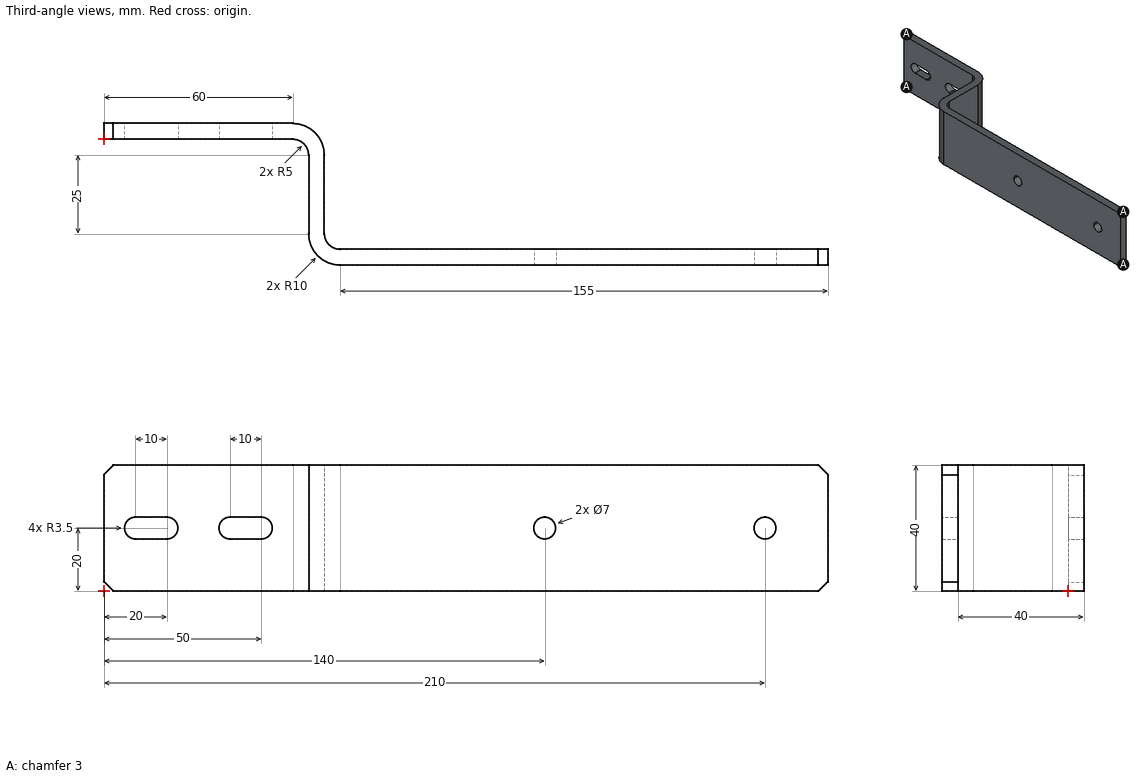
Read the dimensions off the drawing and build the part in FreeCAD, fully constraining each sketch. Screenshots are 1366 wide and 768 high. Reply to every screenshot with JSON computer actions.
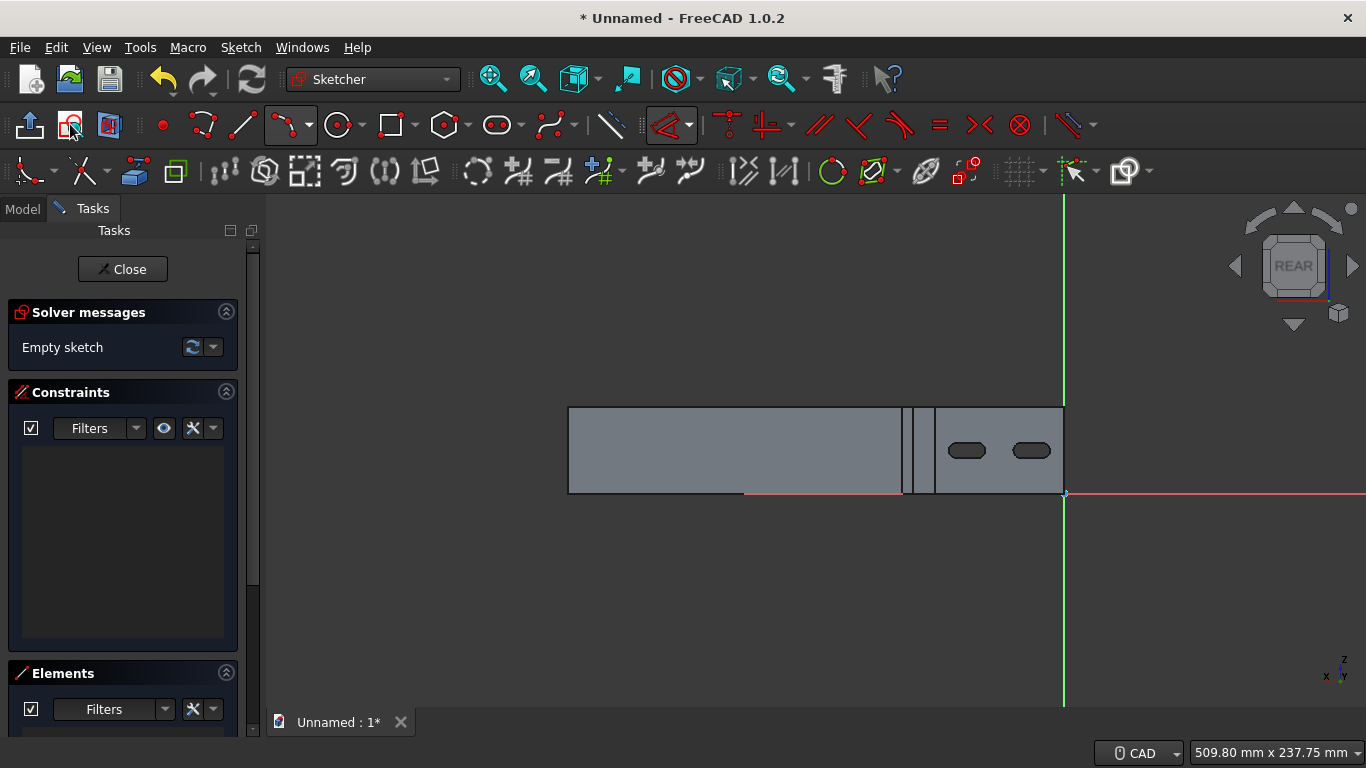
{"action": "left_click", "coordinate": [110, 126]}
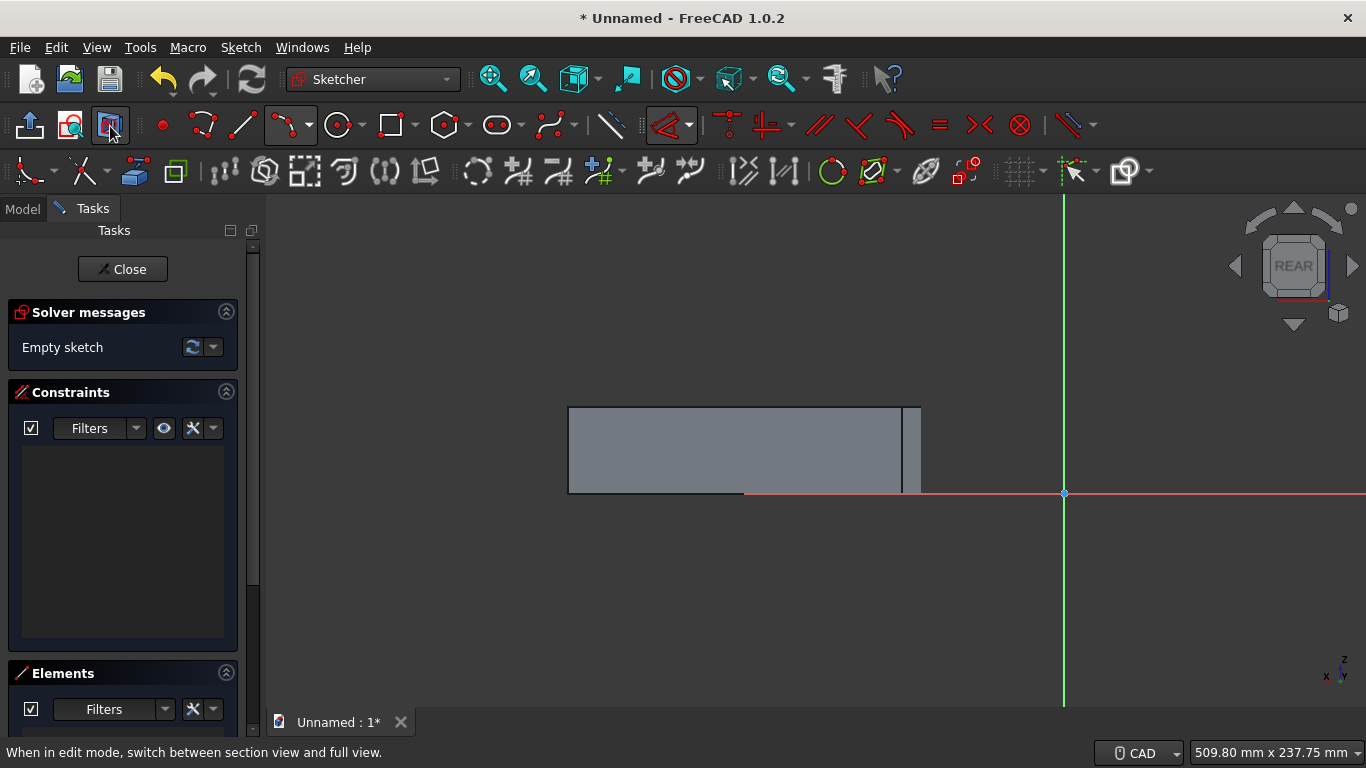
{"action": "scroll", "coordinate": [667, 451], "scroll_direction": "up", "scroll_amount": 7}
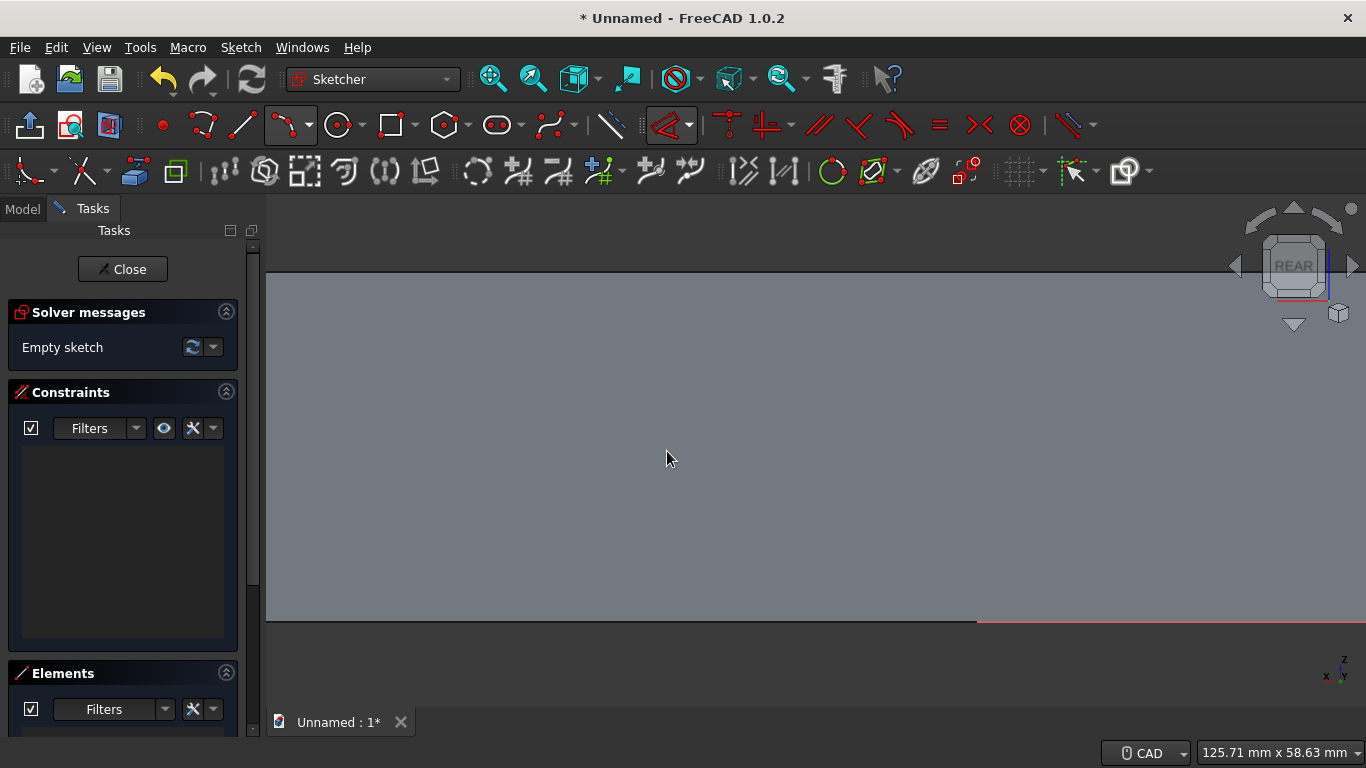
{"action": "left_click", "coordinate": [338, 126]}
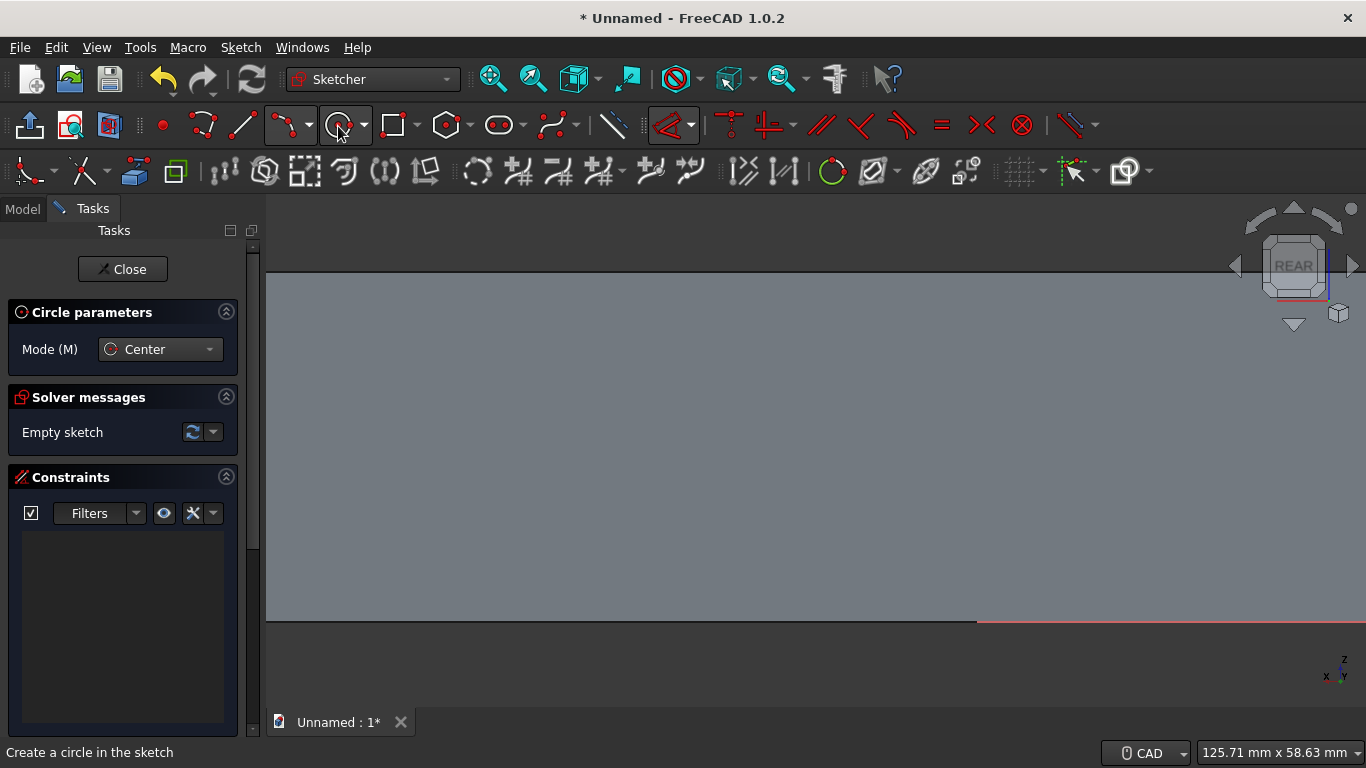
{"action": "left_click", "coordinate": [1051, 447]}
{"action": "mouse_move", "coordinate": [1073, 426]}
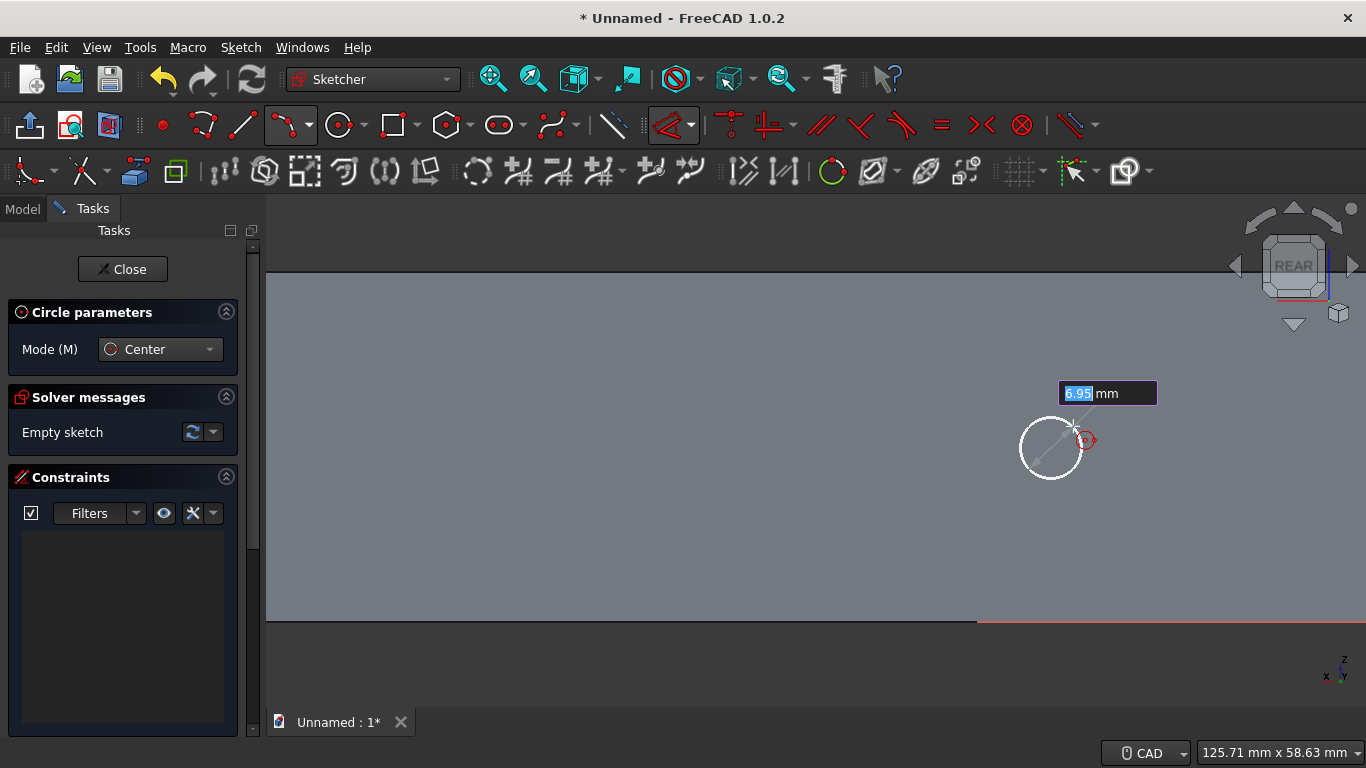
{"action": "type", "text": "7"}
{"action": "key", "text": "Return"}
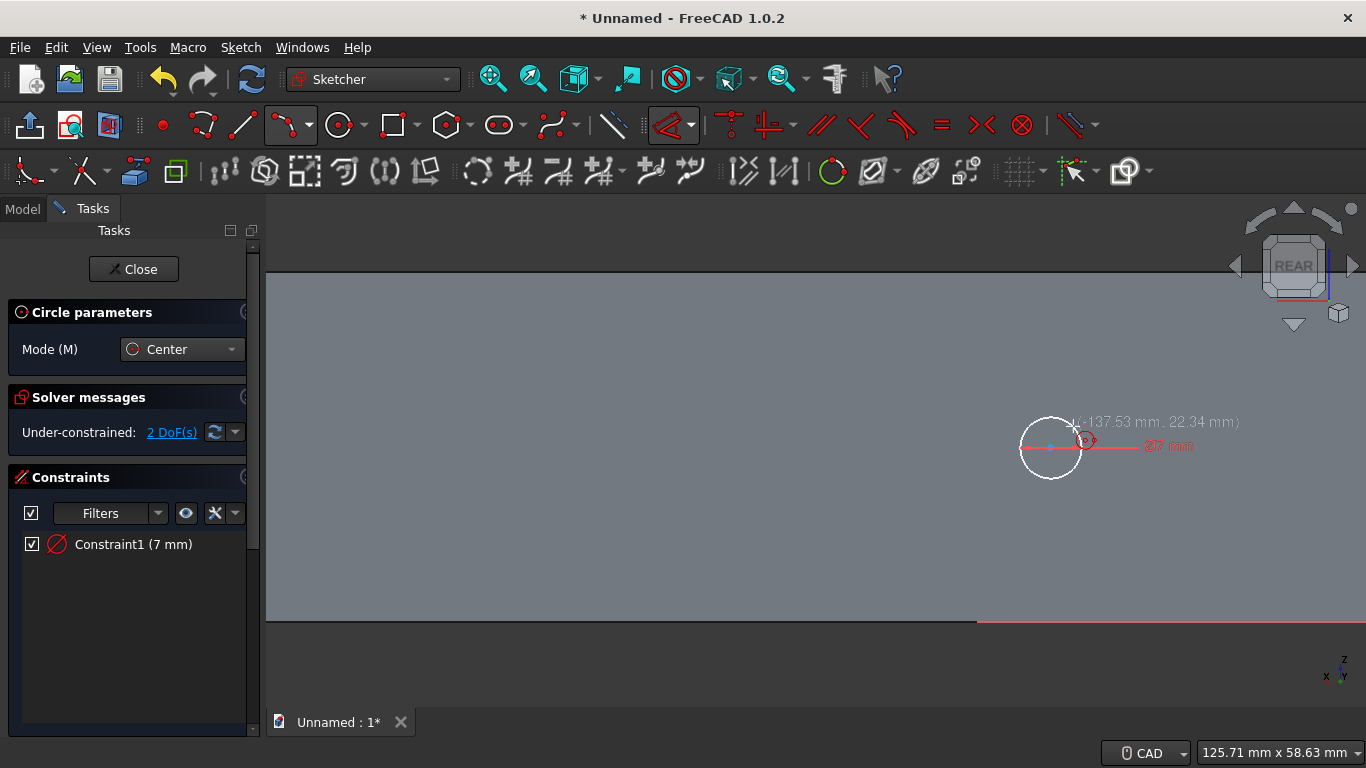
{"action": "left_click", "coordinate": [439, 447]}
{"action": "mouse_move", "coordinate": [461, 426]}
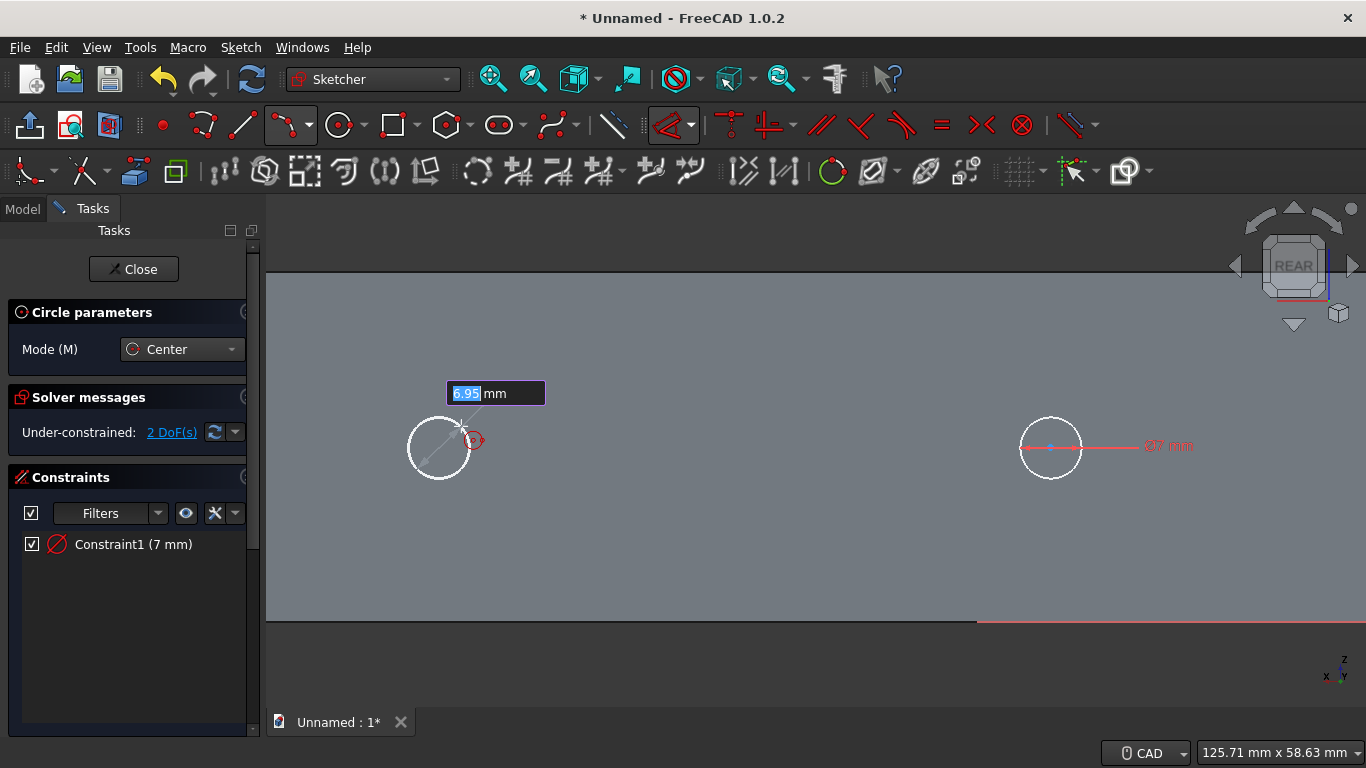
{"action": "type", "text": "7"}
{"action": "key", "text": "Return"}
{"action": "key", "text": "Escape"}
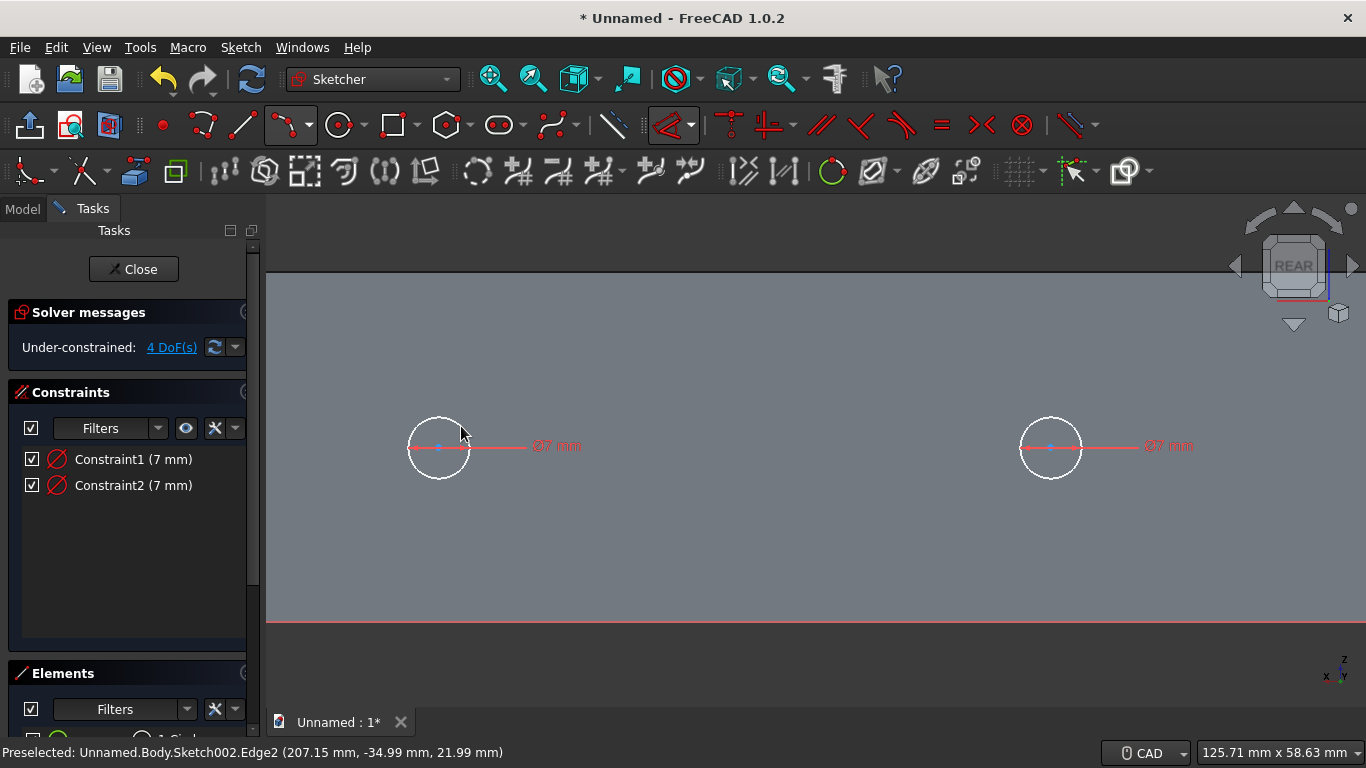
{"action": "left_click", "coordinate": [1051, 448]}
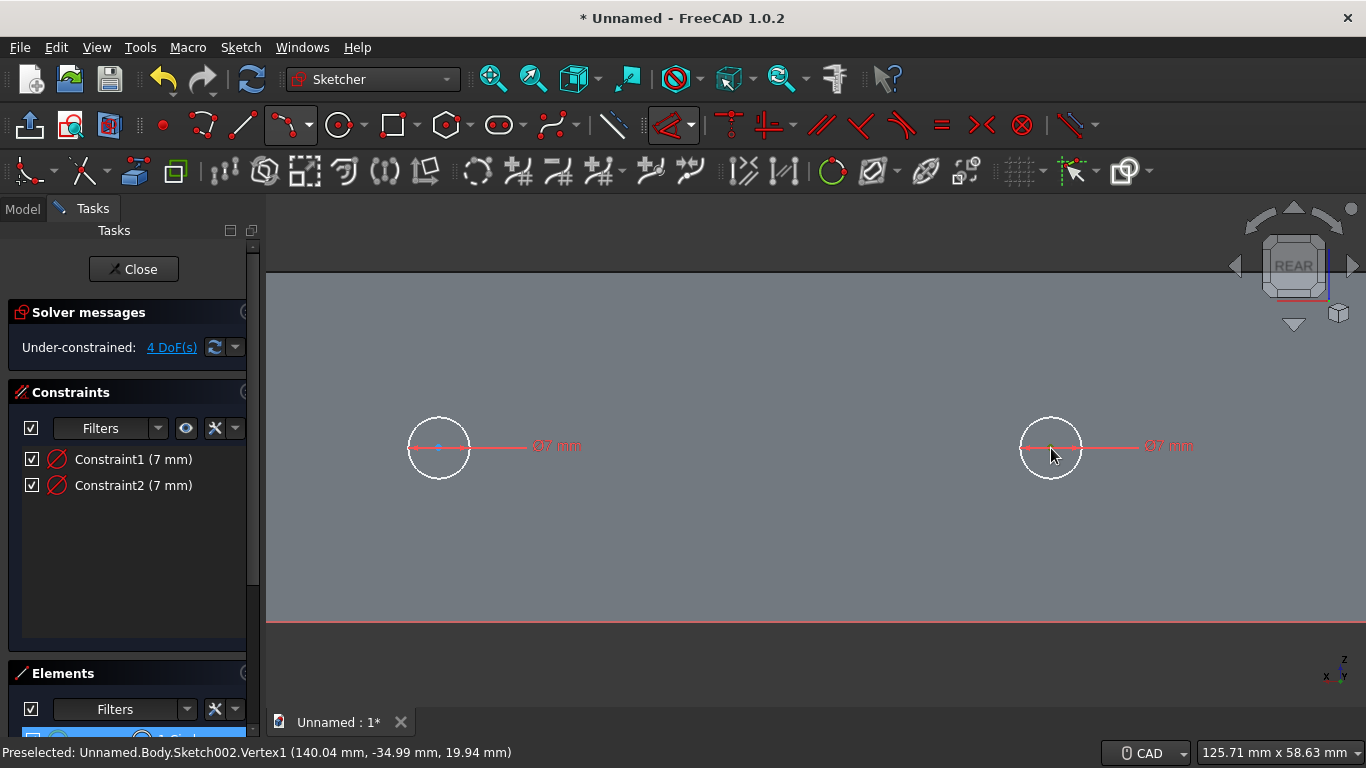
{"action": "left_click", "coordinate": [439, 448]}